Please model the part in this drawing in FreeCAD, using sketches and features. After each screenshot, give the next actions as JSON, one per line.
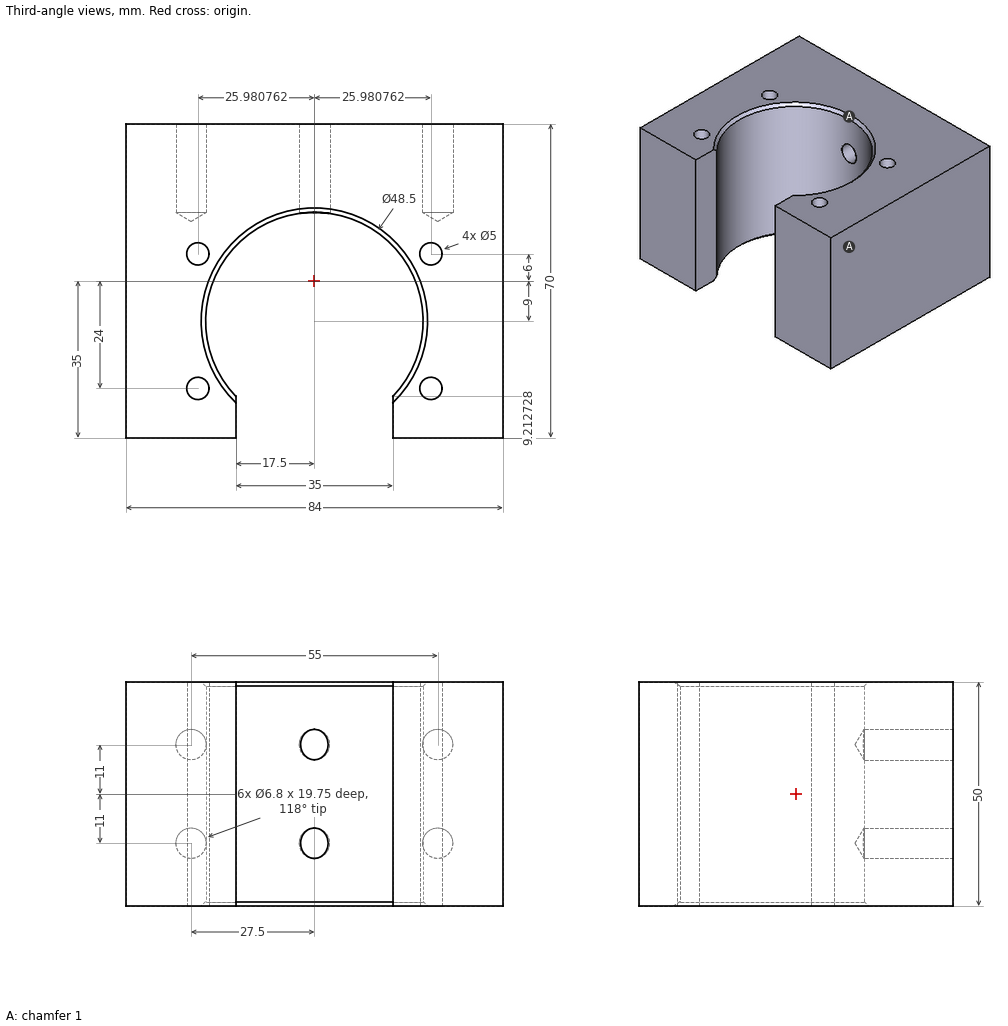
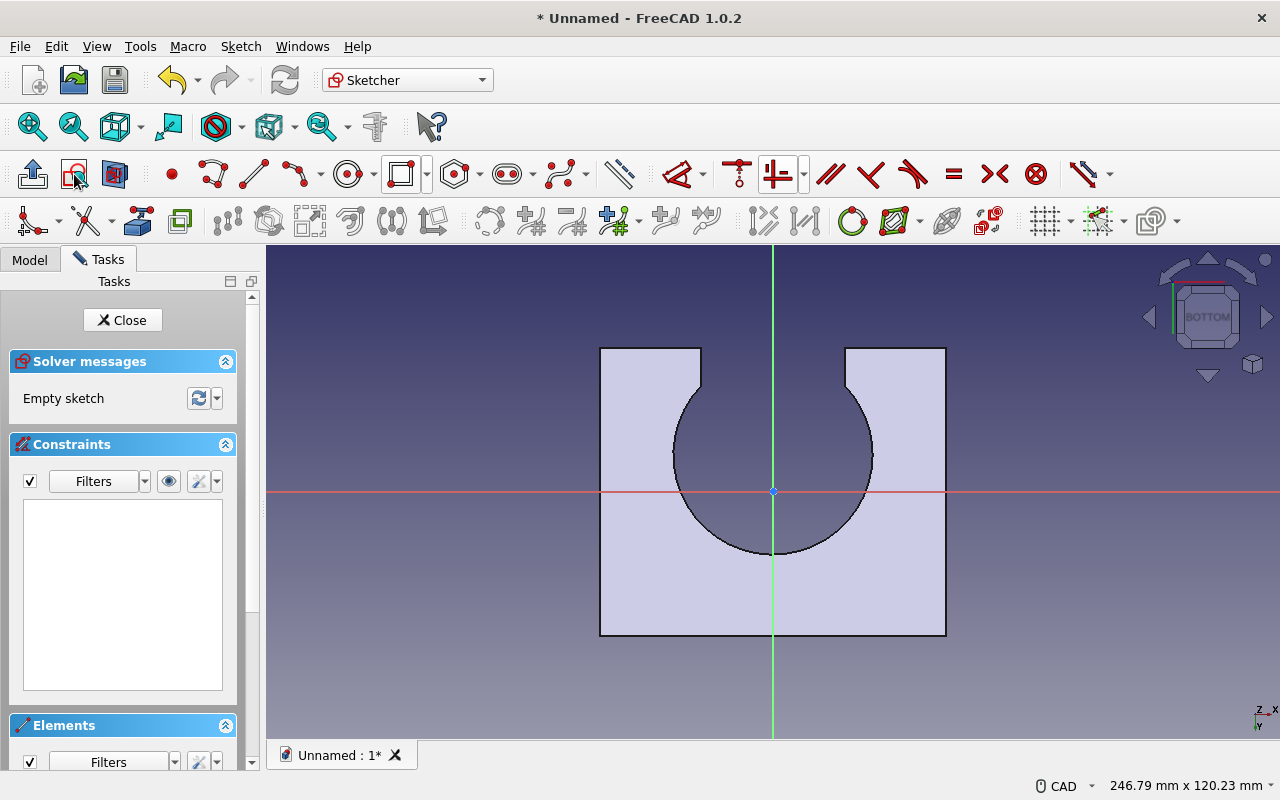
{"action": "scroll", "coordinate": [829, 425], "scroll_direction": "up", "scroll_amount": 4}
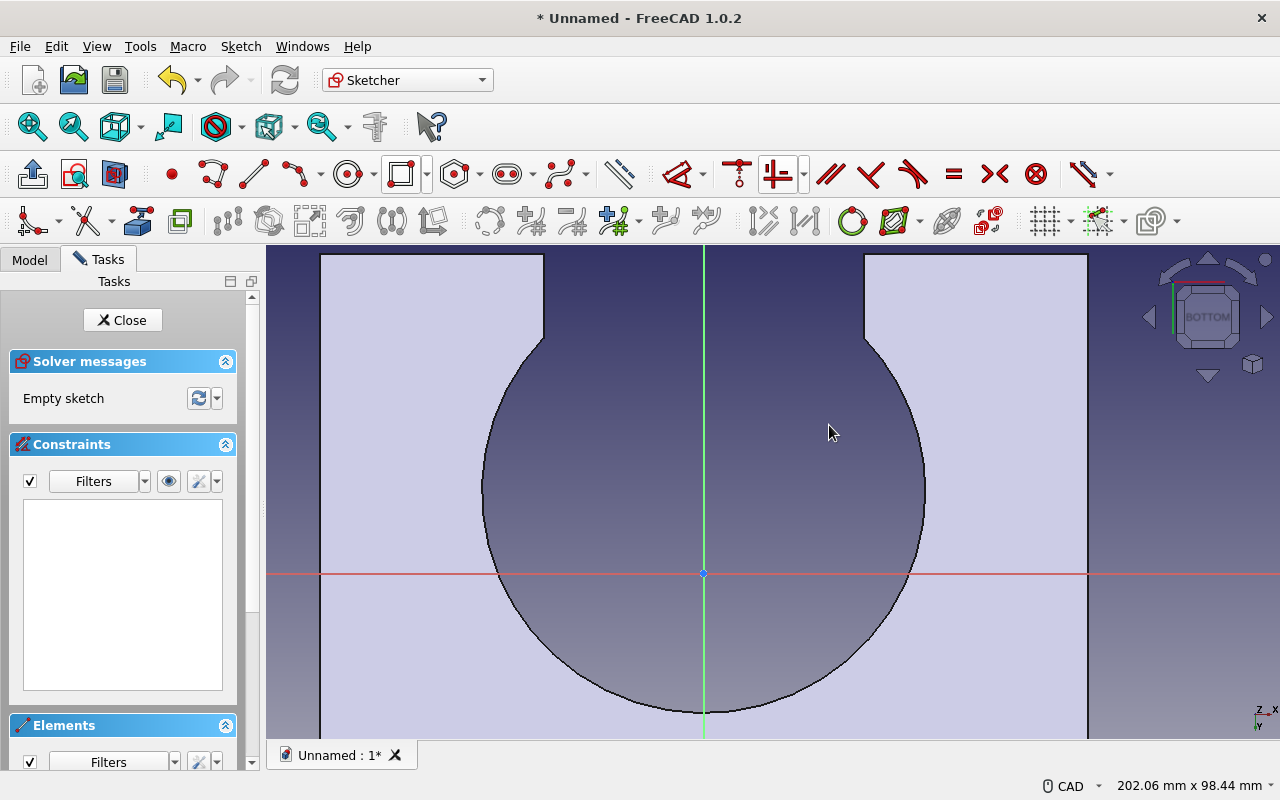
{"action": "left_click", "coordinate": [348, 174]}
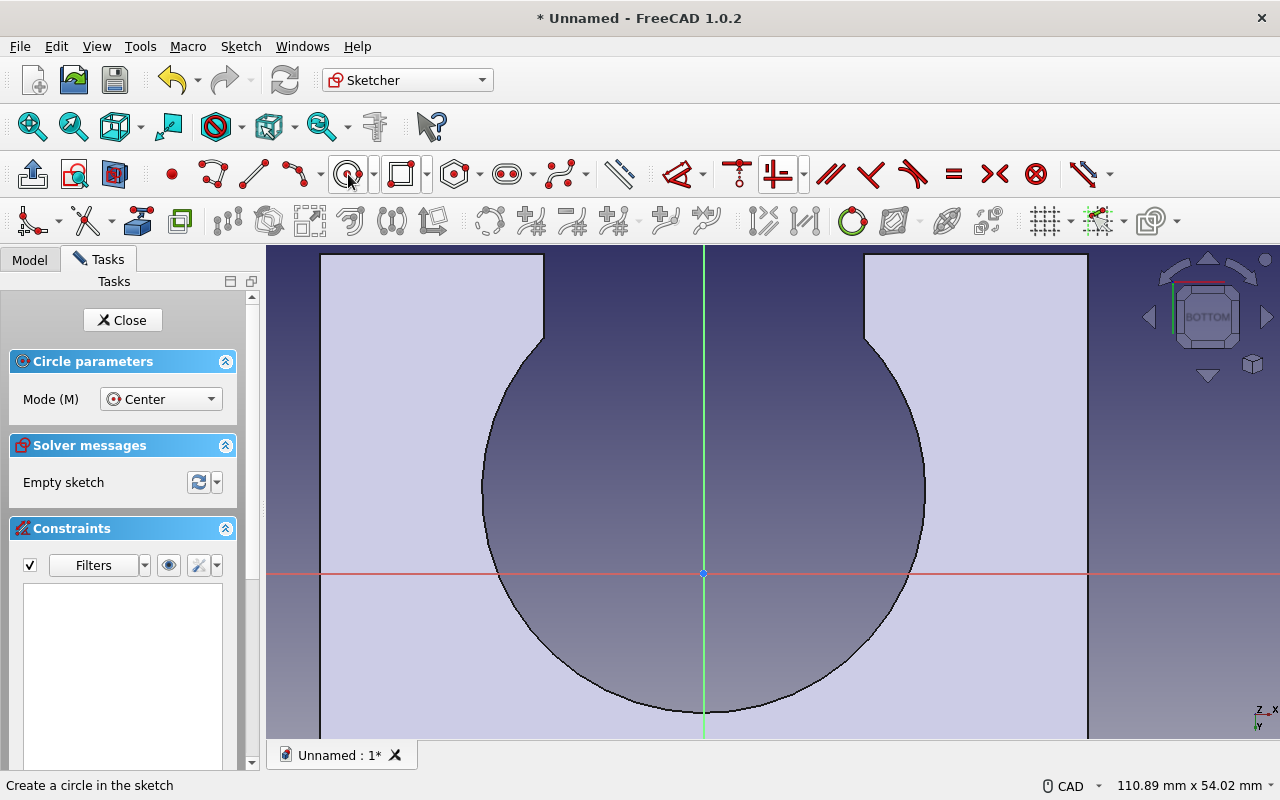
{"action": "left_click", "coordinate": [941, 629]}
{"action": "mouse_move", "coordinate": [957, 612]}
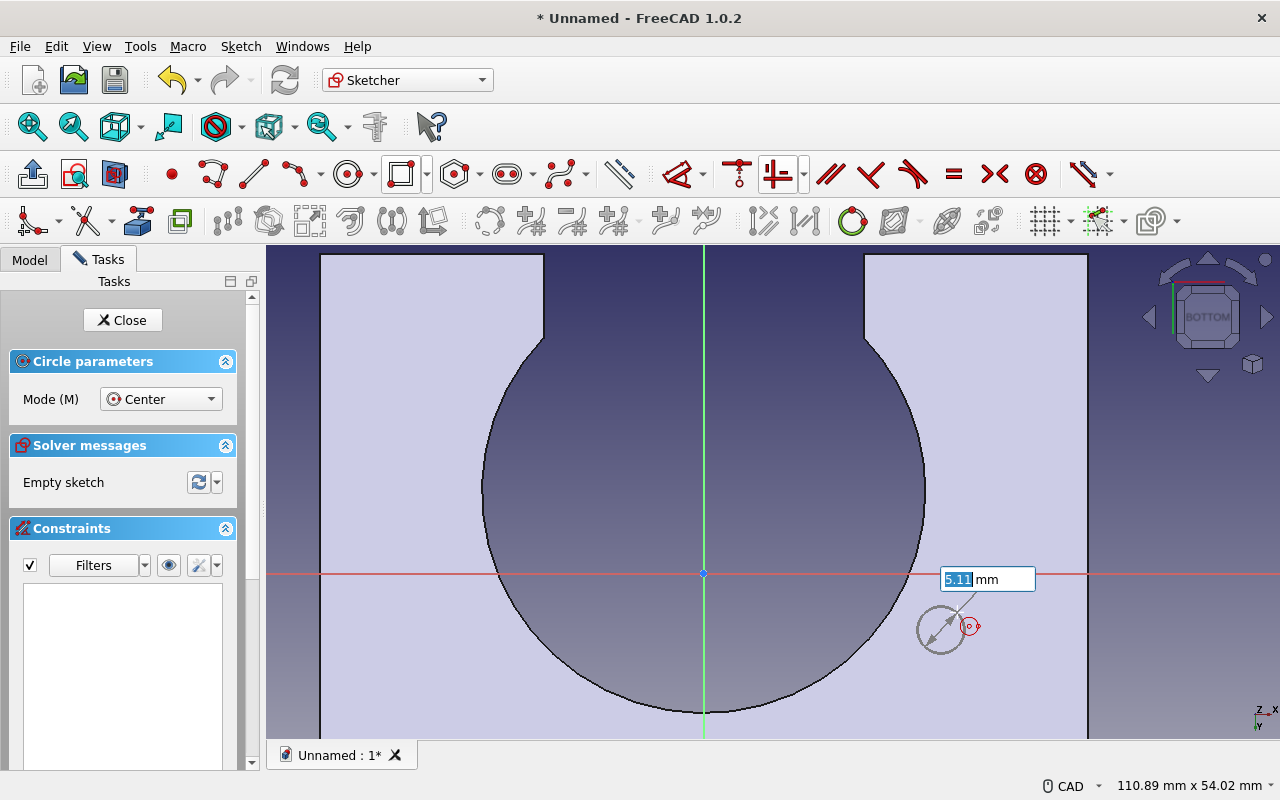
{"action": "type", "text": "5"}
{"action": "key", "text": "Return"}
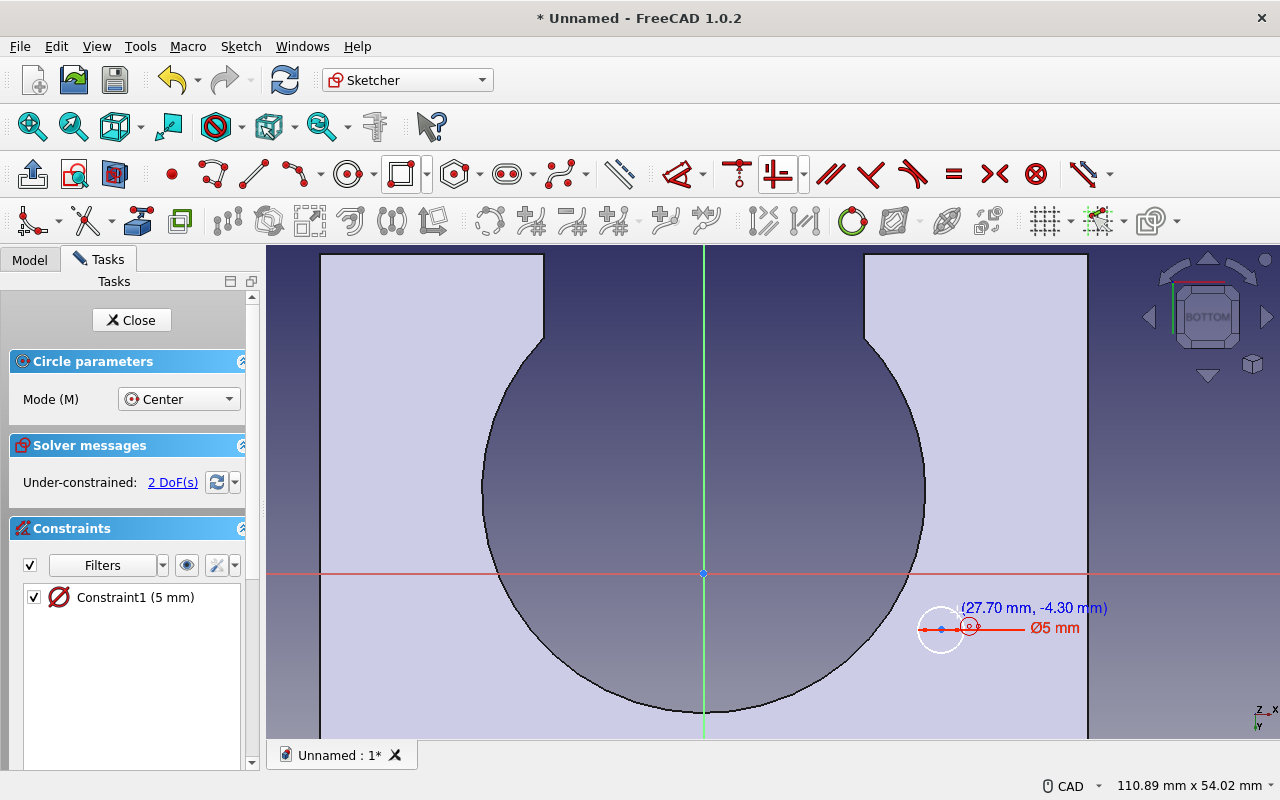
{"action": "left_click", "coordinate": [466, 629]}
{"action": "mouse_move", "coordinate": [482, 612]}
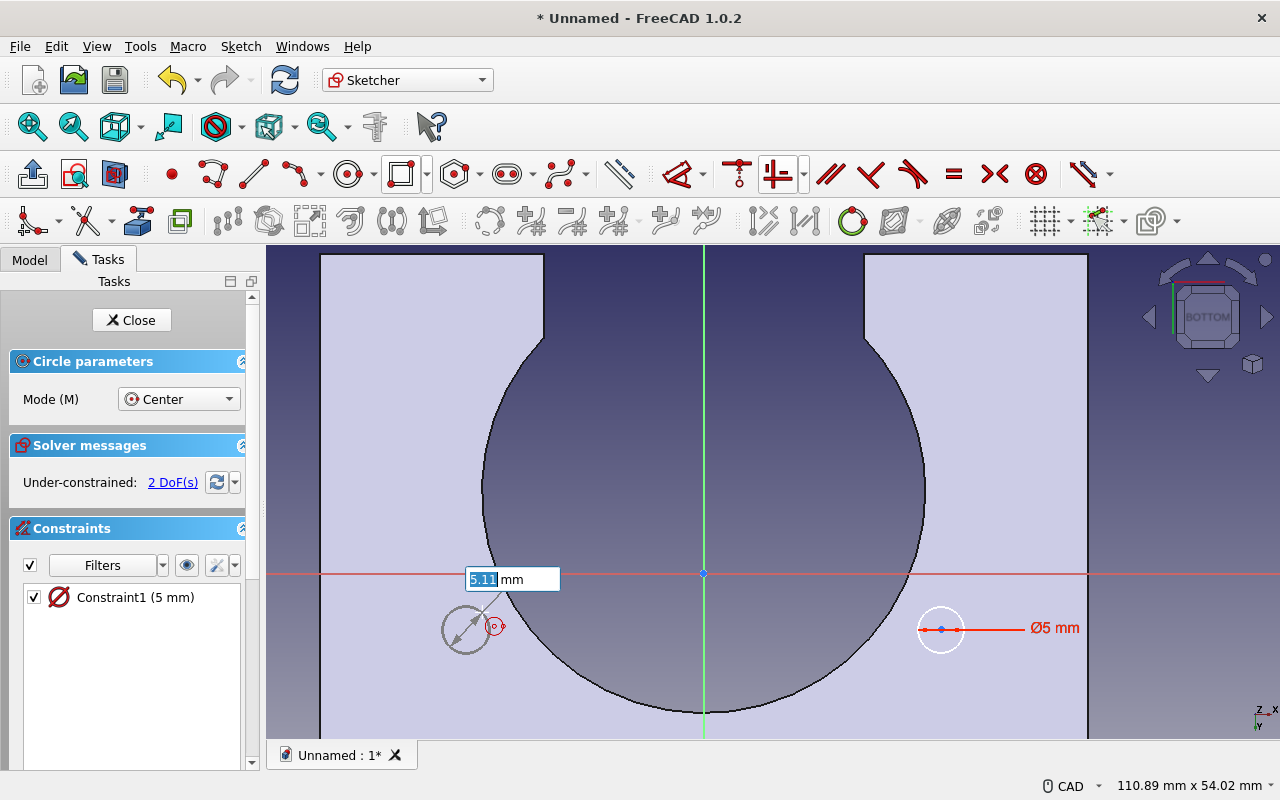
{"action": "type", "text": "5"}
{"action": "key", "text": "Return"}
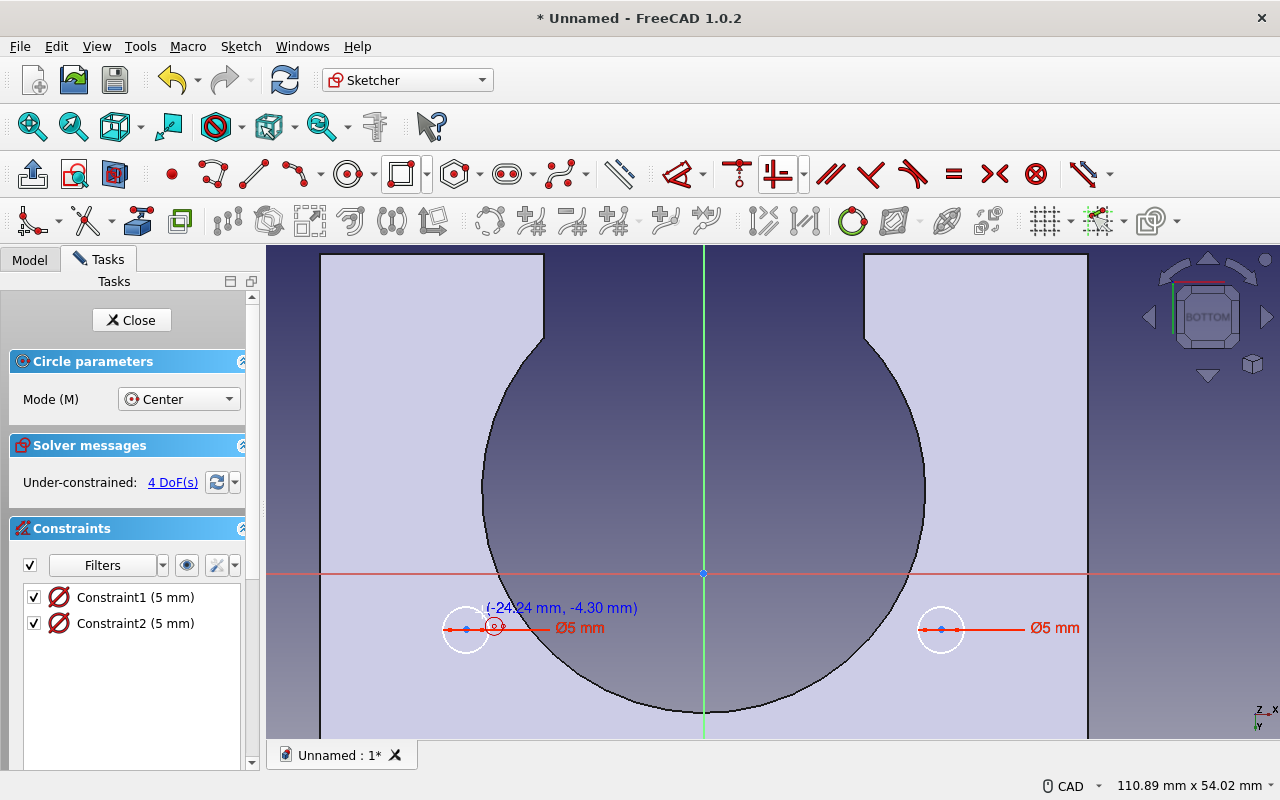
{"action": "left_click", "coordinate": [466, 354]}
{"action": "mouse_move", "coordinate": [482, 338]}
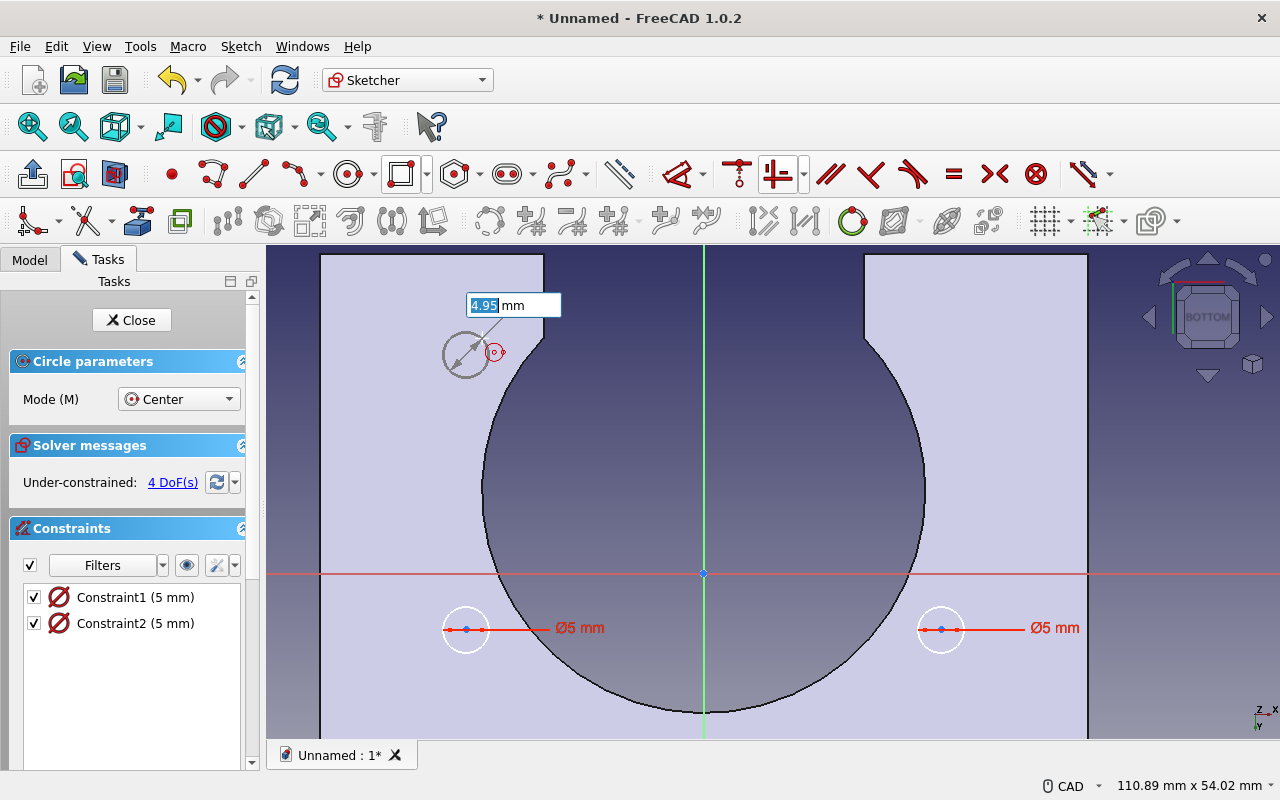
{"action": "type", "text": "5"}
{"action": "key", "text": "Return"}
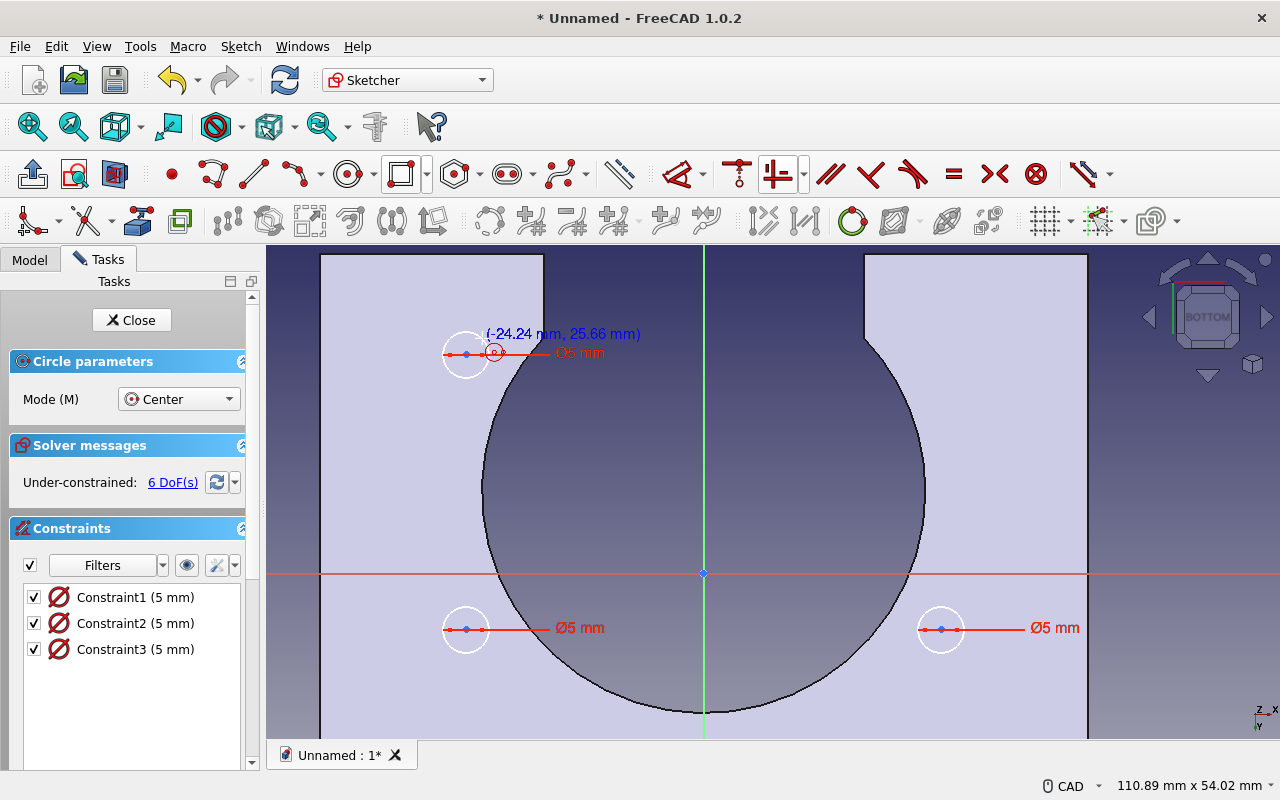
{"action": "left_click", "coordinate": [941, 354]}
{"action": "mouse_move", "coordinate": [957, 338]}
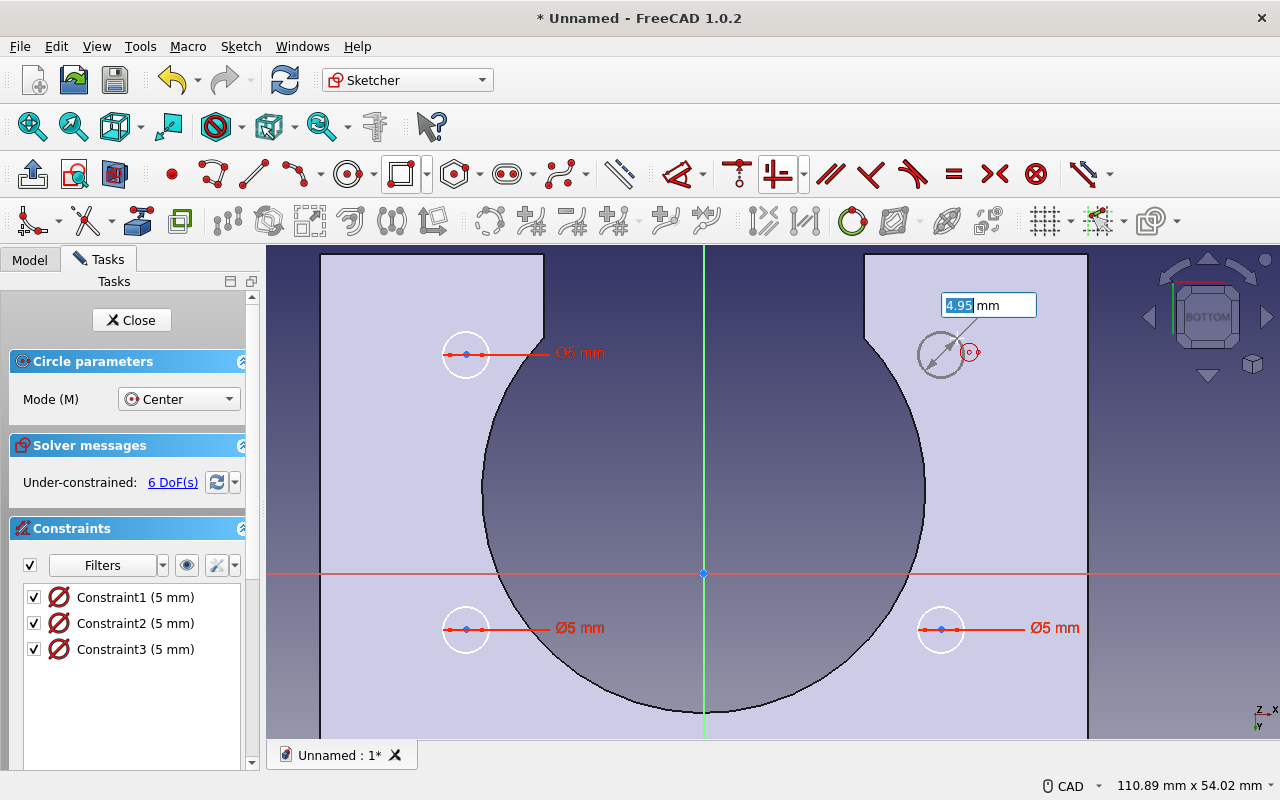
{"action": "type", "text": "5"}
{"action": "key", "text": "Return"}
{"action": "key", "text": "Escape"}